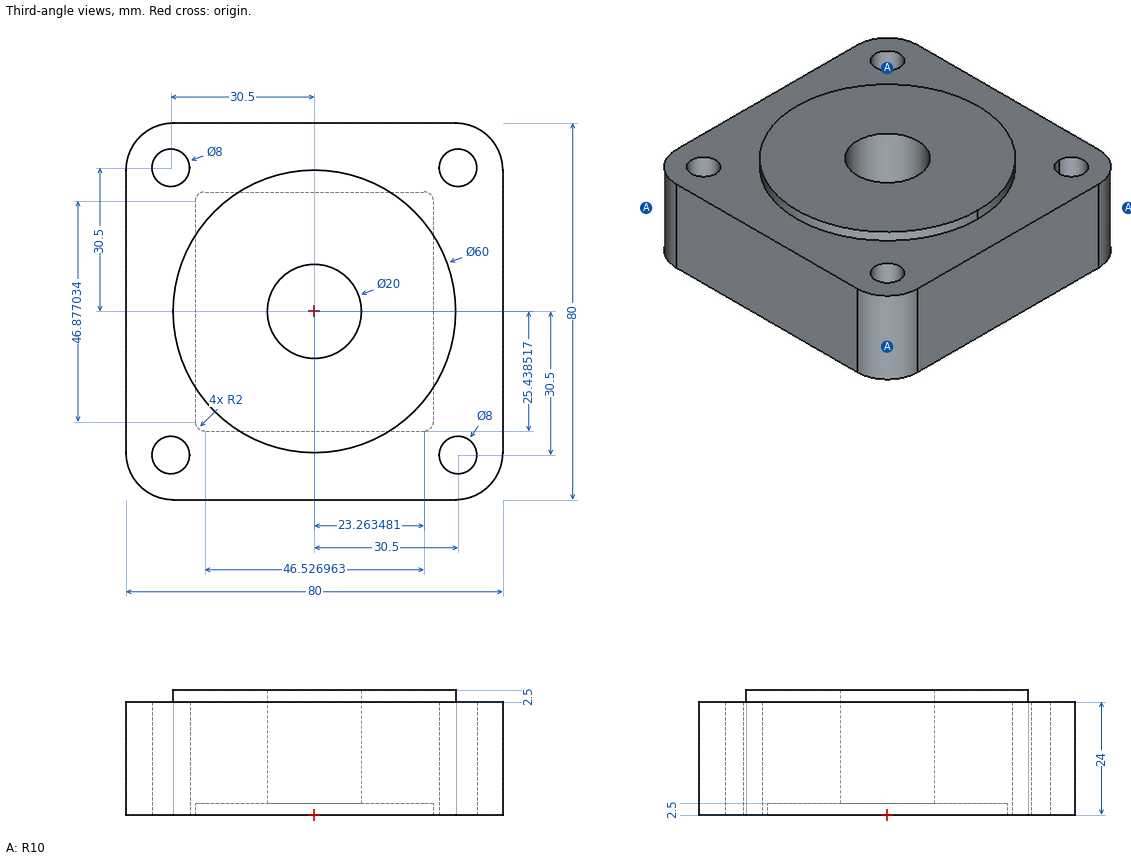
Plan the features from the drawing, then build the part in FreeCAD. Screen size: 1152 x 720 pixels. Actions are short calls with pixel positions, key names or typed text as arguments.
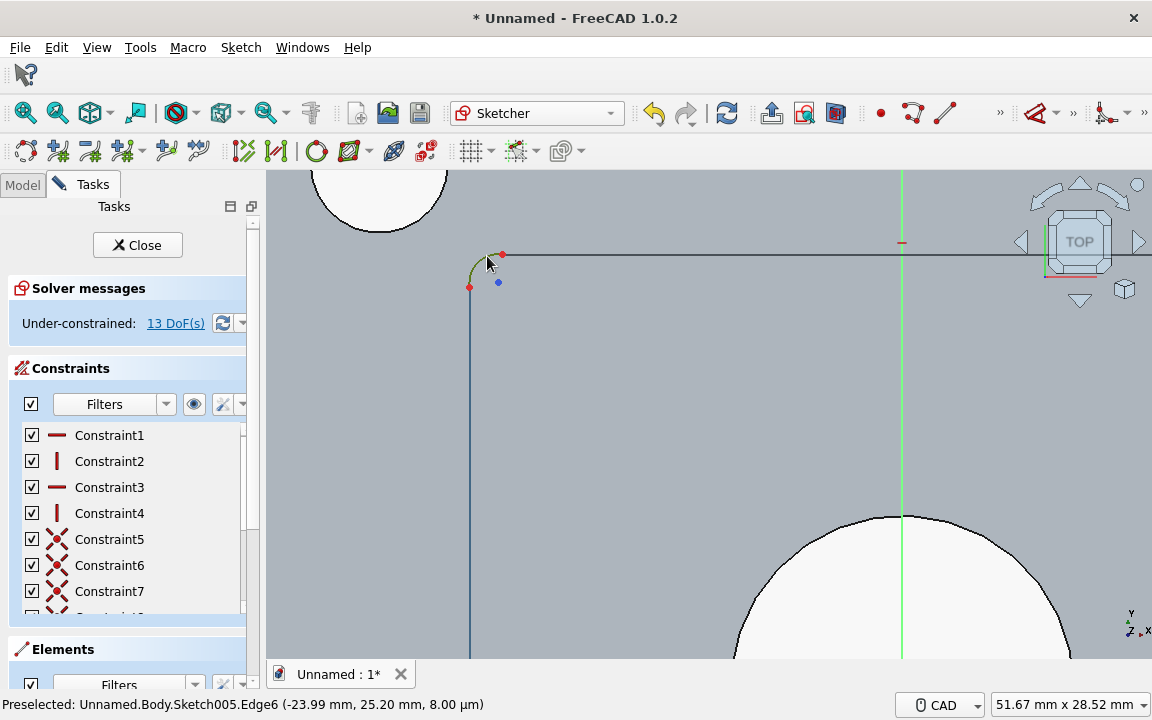
key(t)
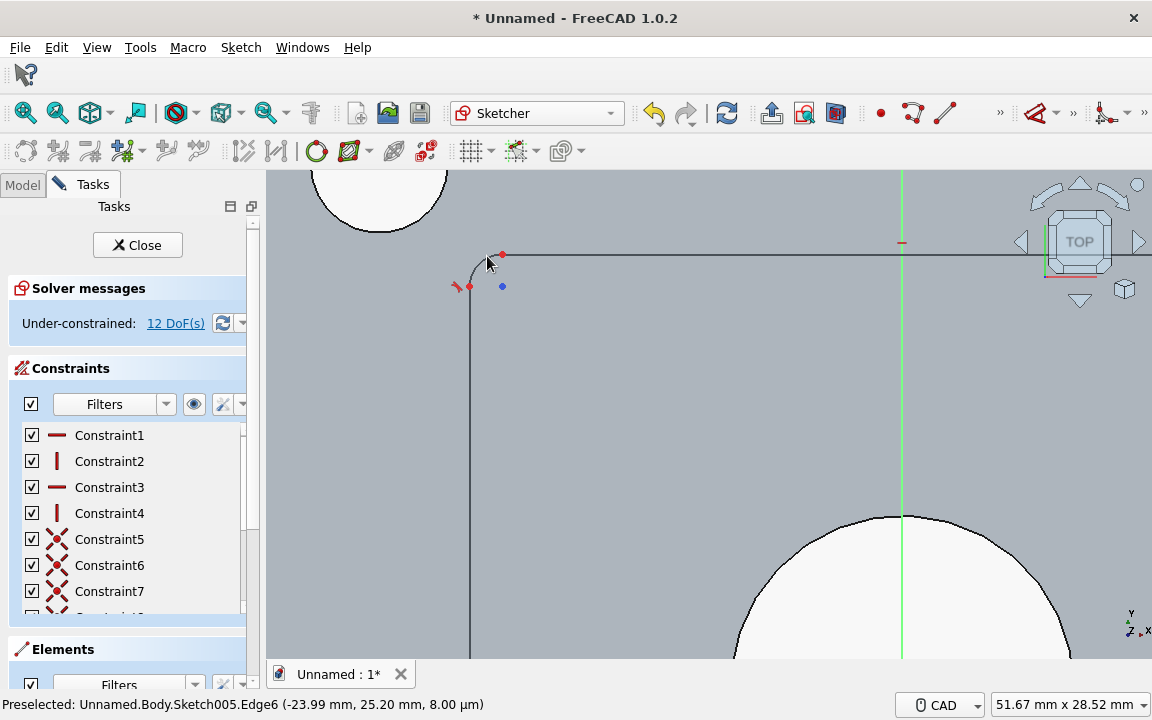
click(742, 255)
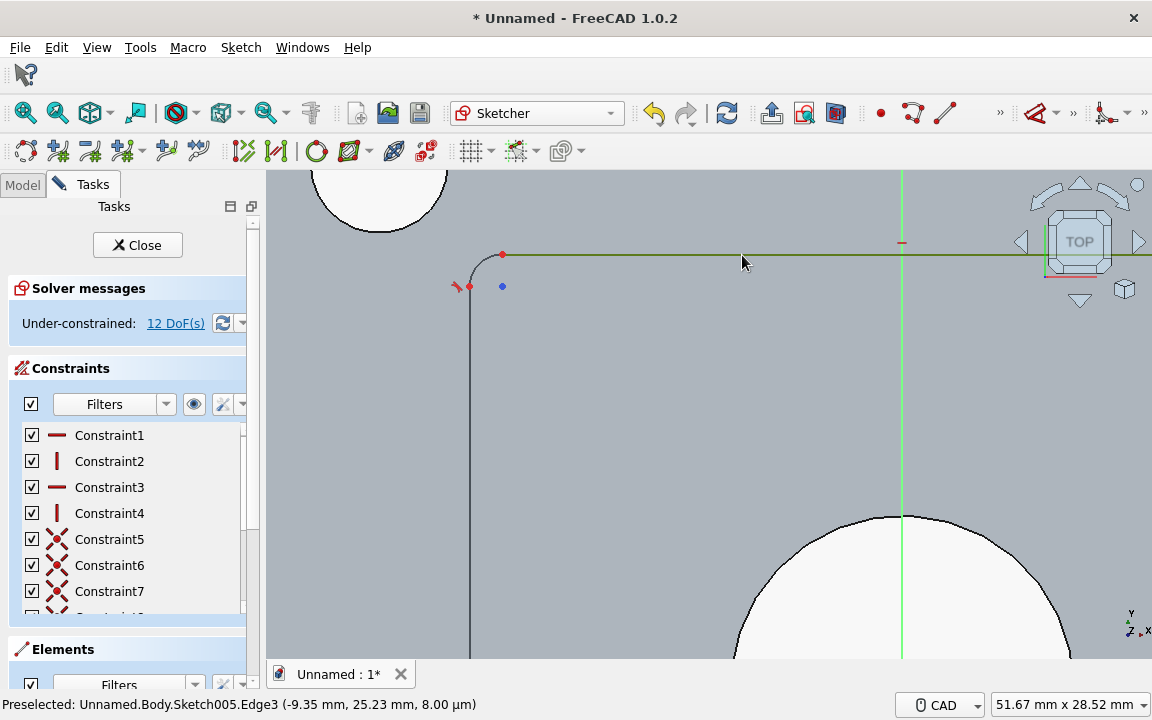
click(488, 258)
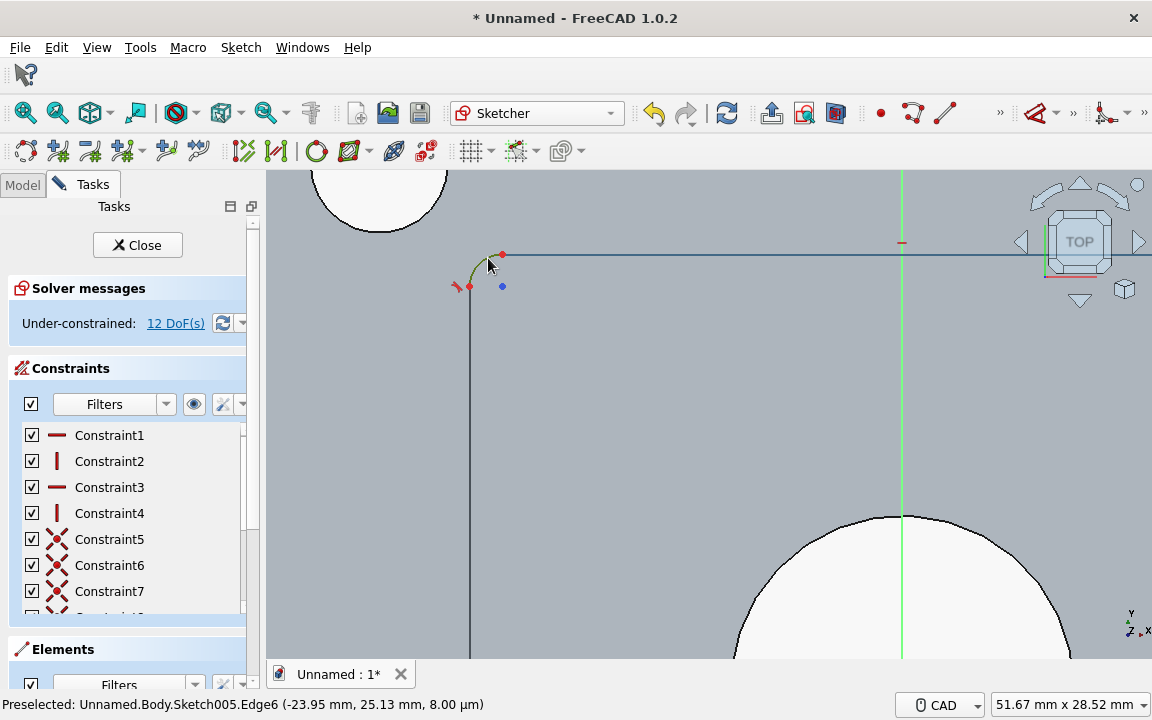
key(t)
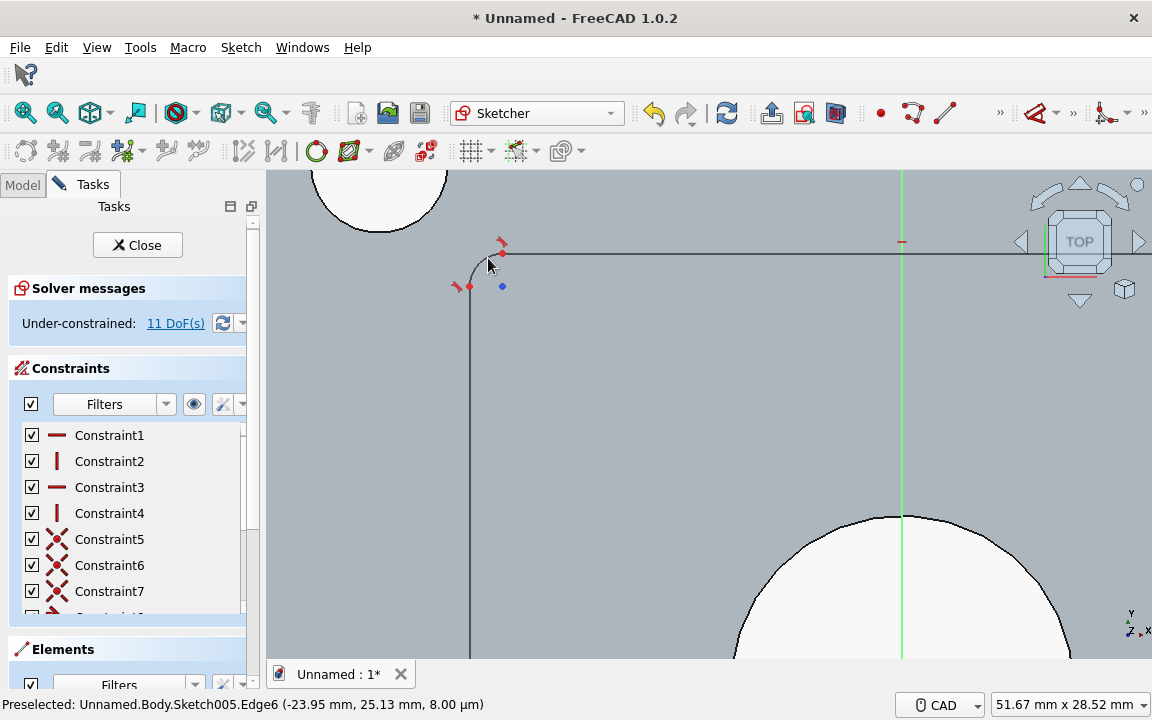
click(742, 254)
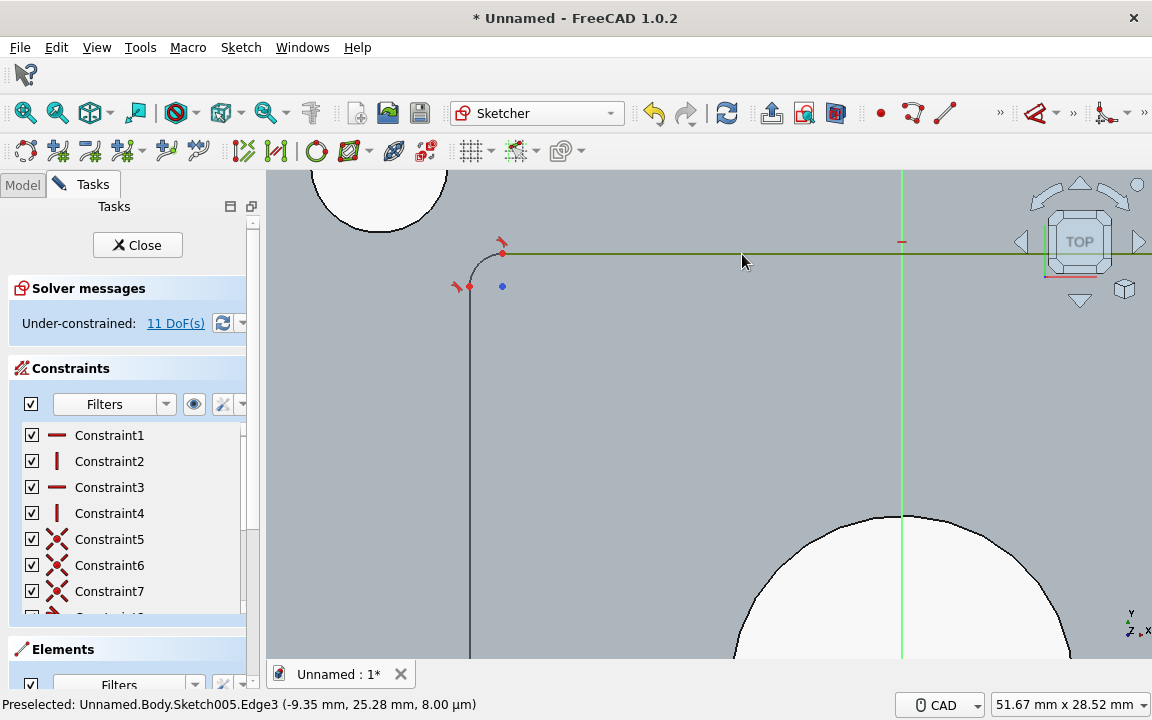
scroll(488, 256, down, 5)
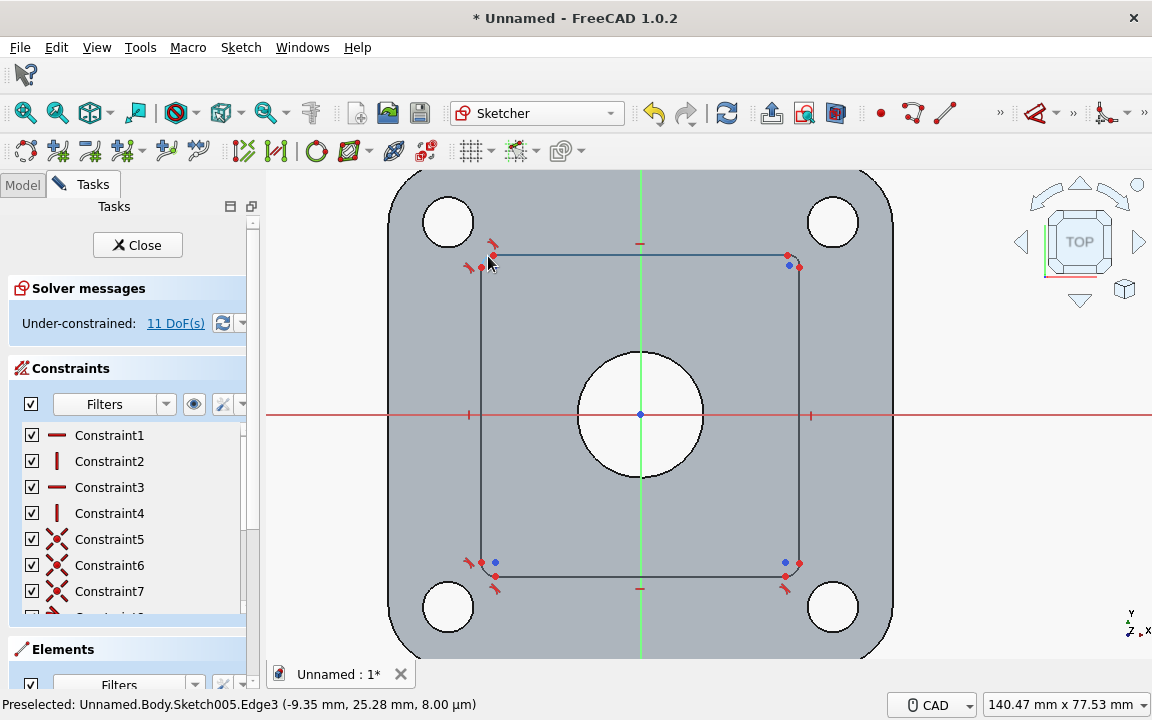
scroll(799, 262, up, 5)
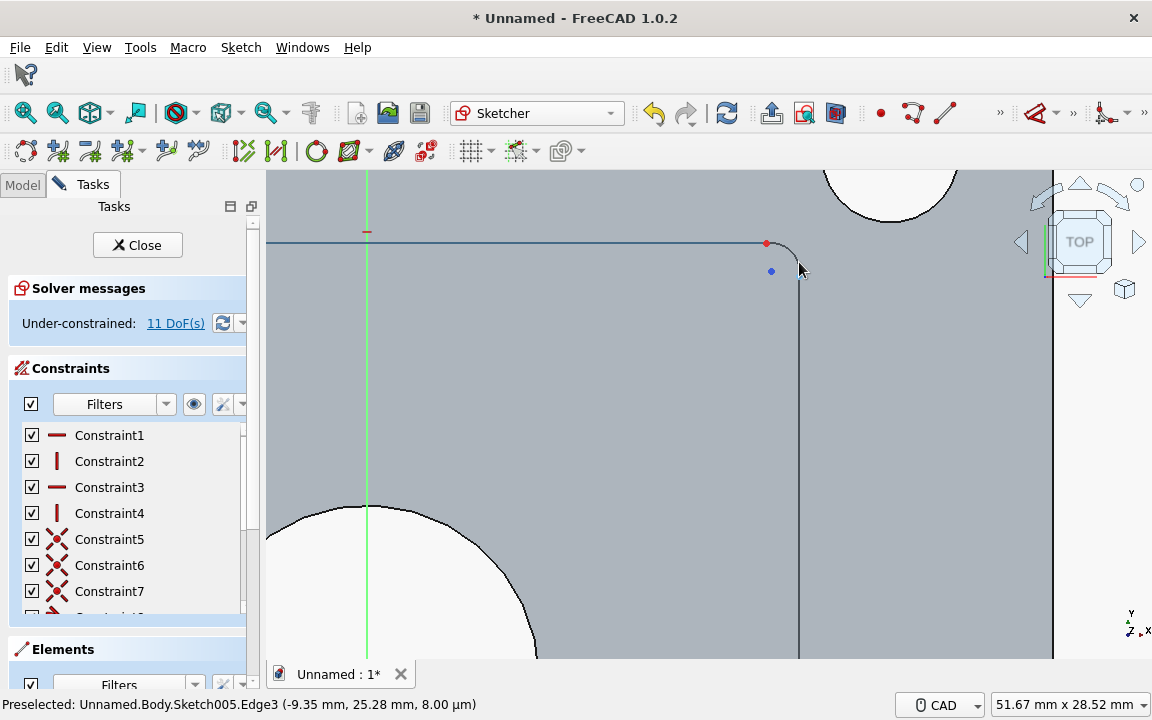
click(798, 261)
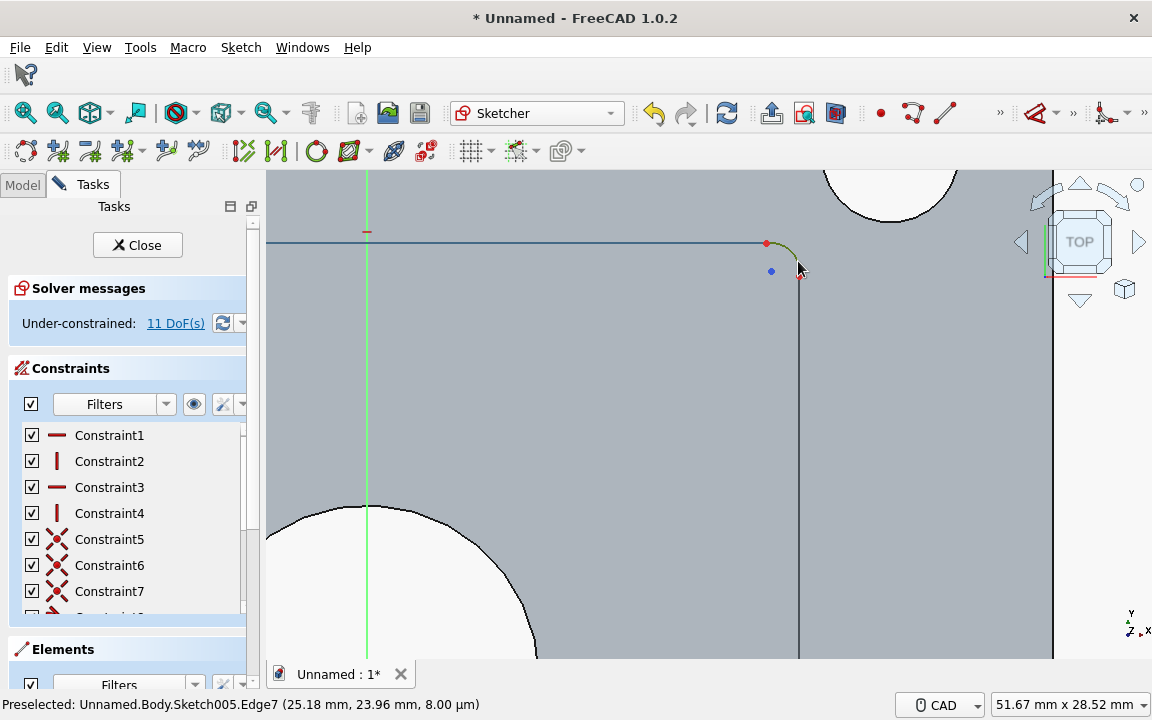
key(t)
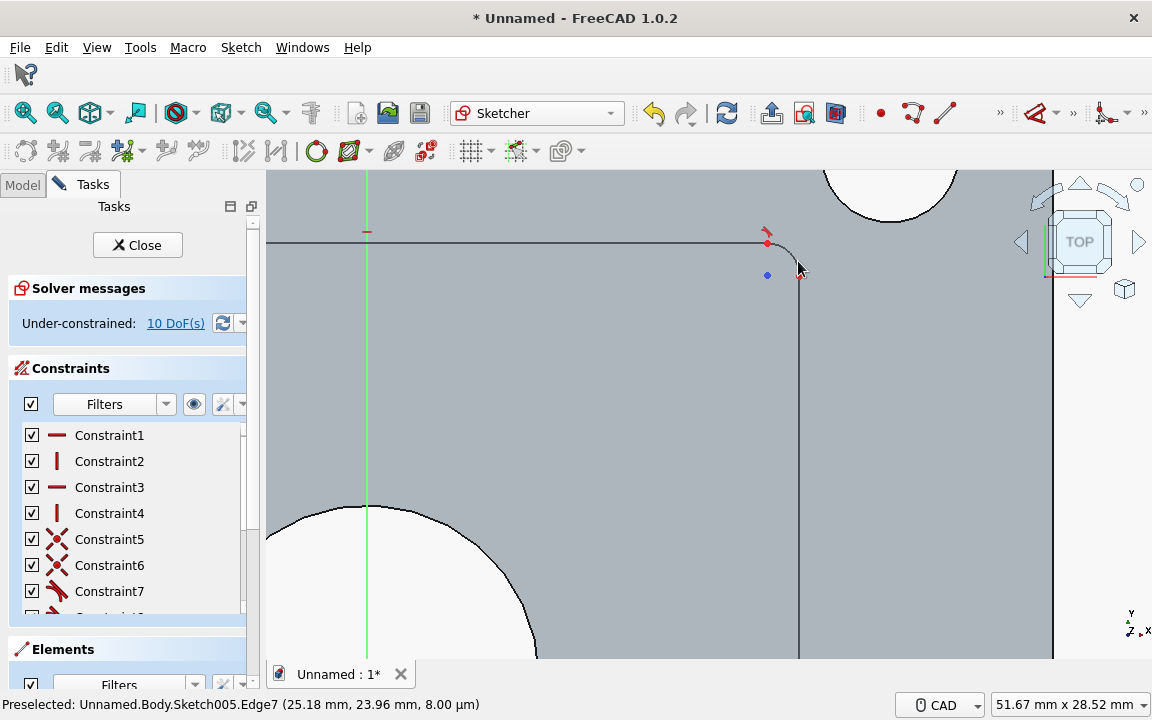
click(799, 518)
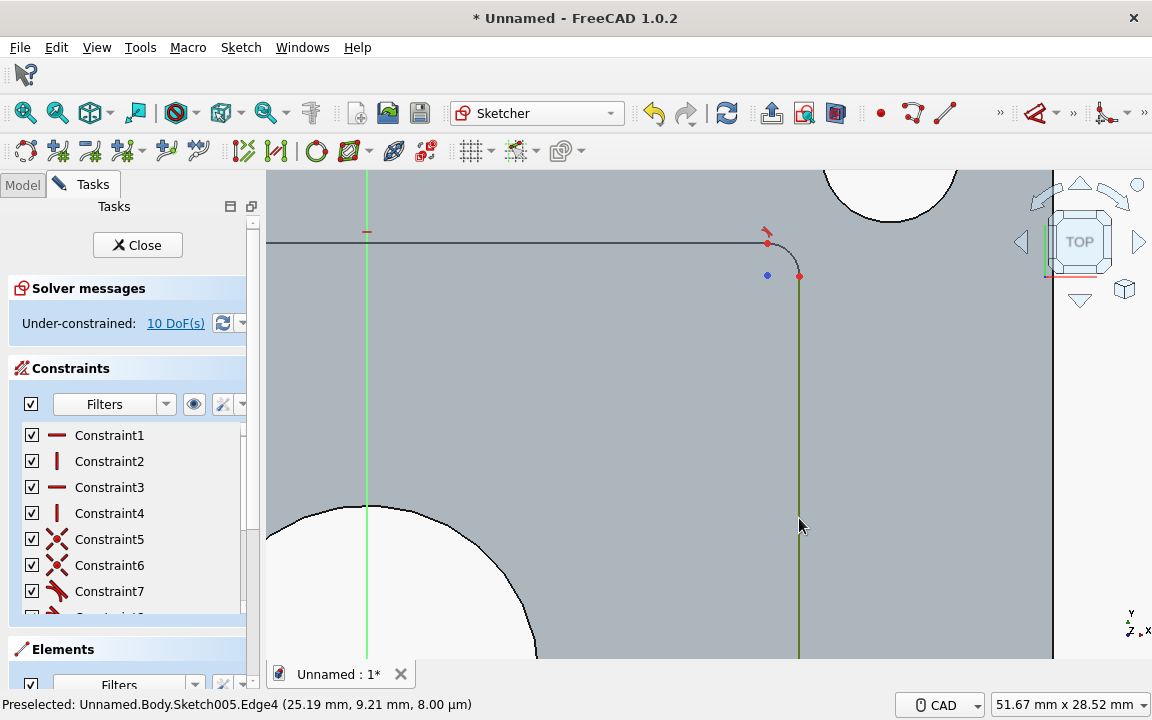
click(796, 262)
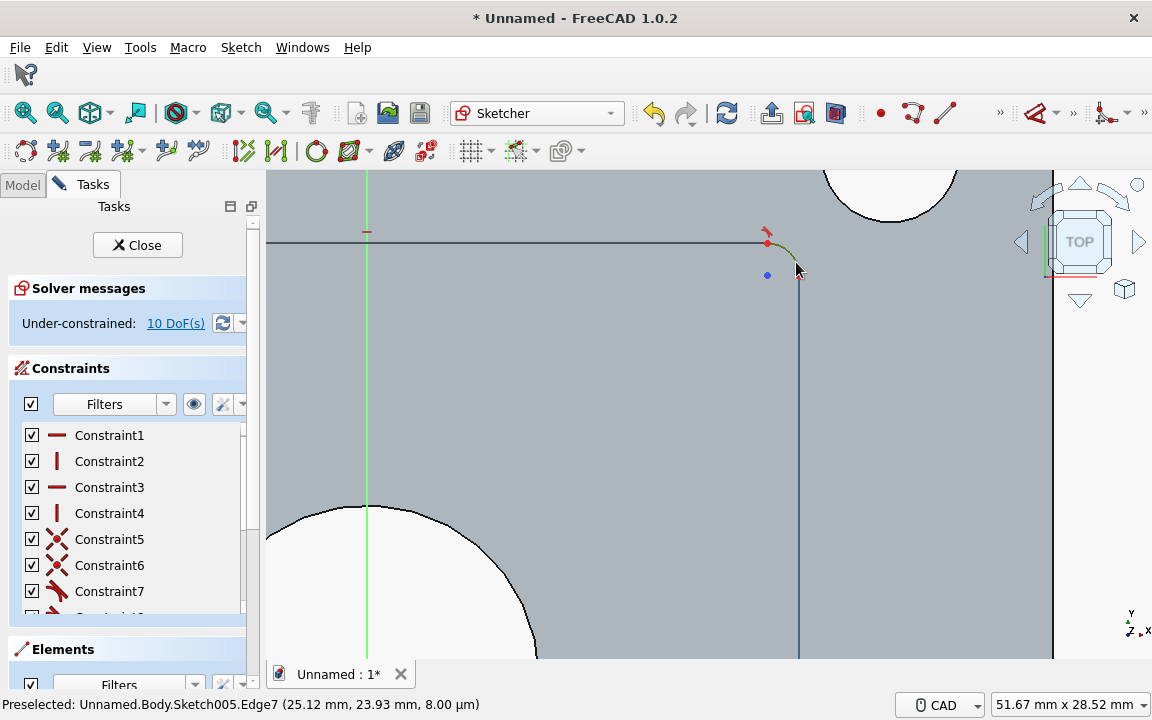
key(t)